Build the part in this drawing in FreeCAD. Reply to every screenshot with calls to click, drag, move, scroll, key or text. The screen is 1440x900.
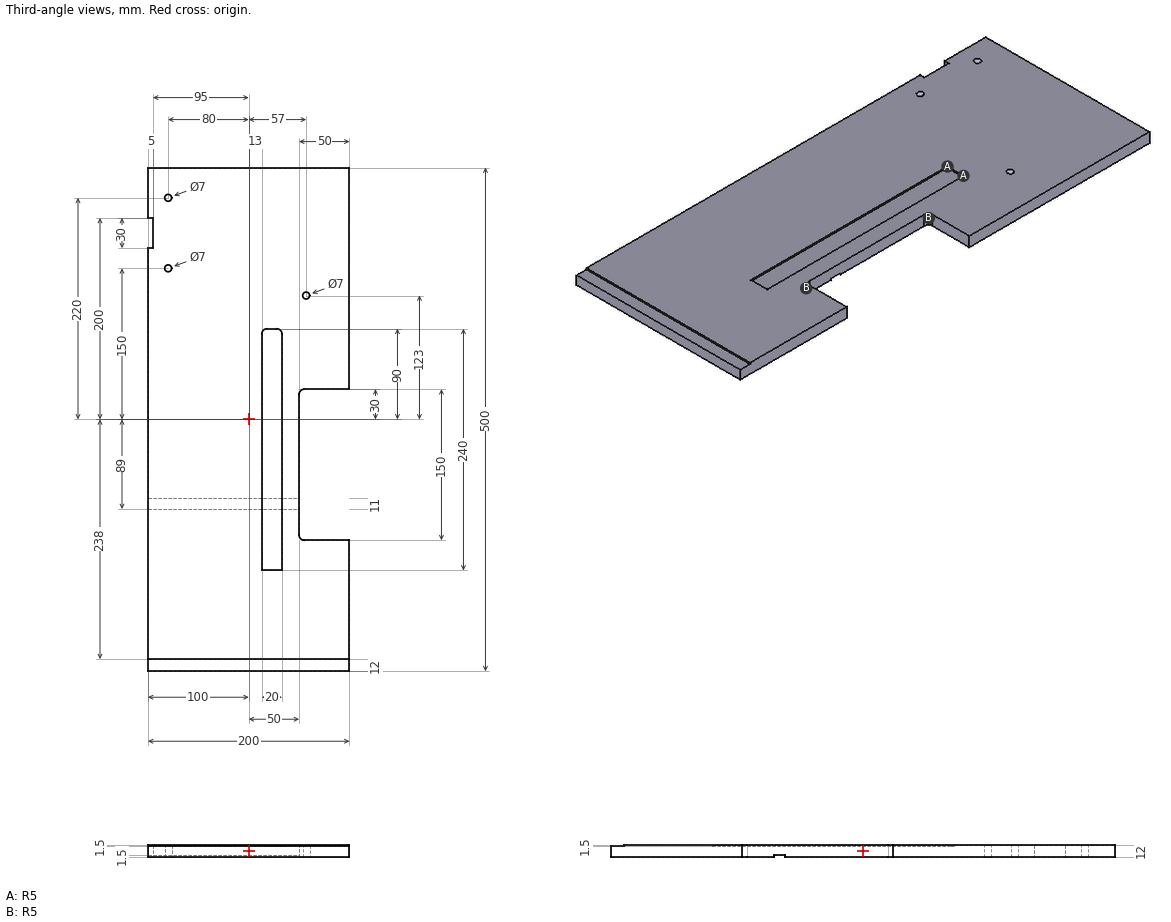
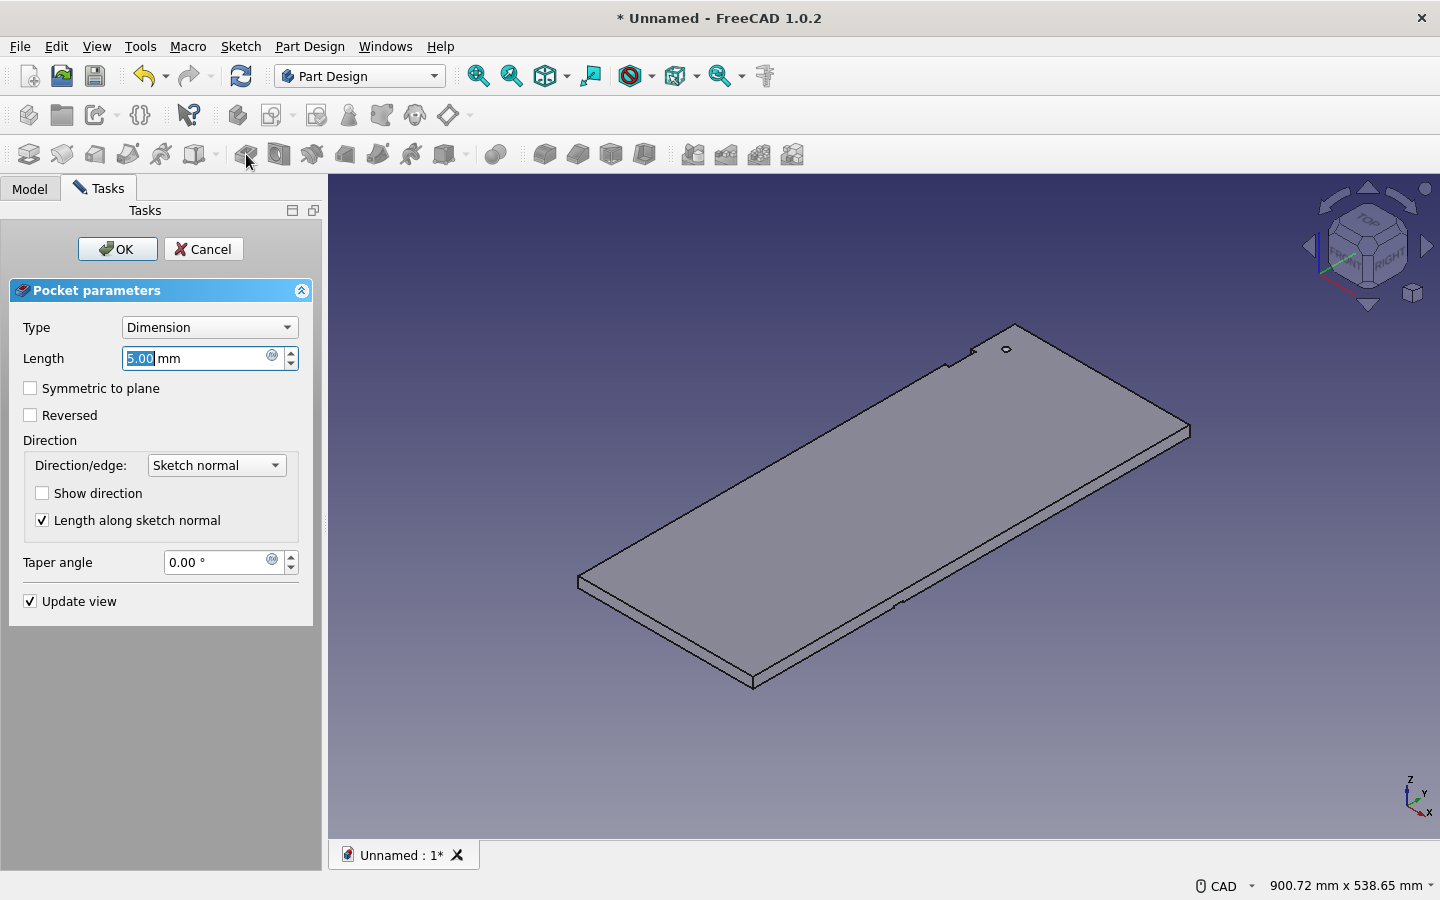
click(210, 328)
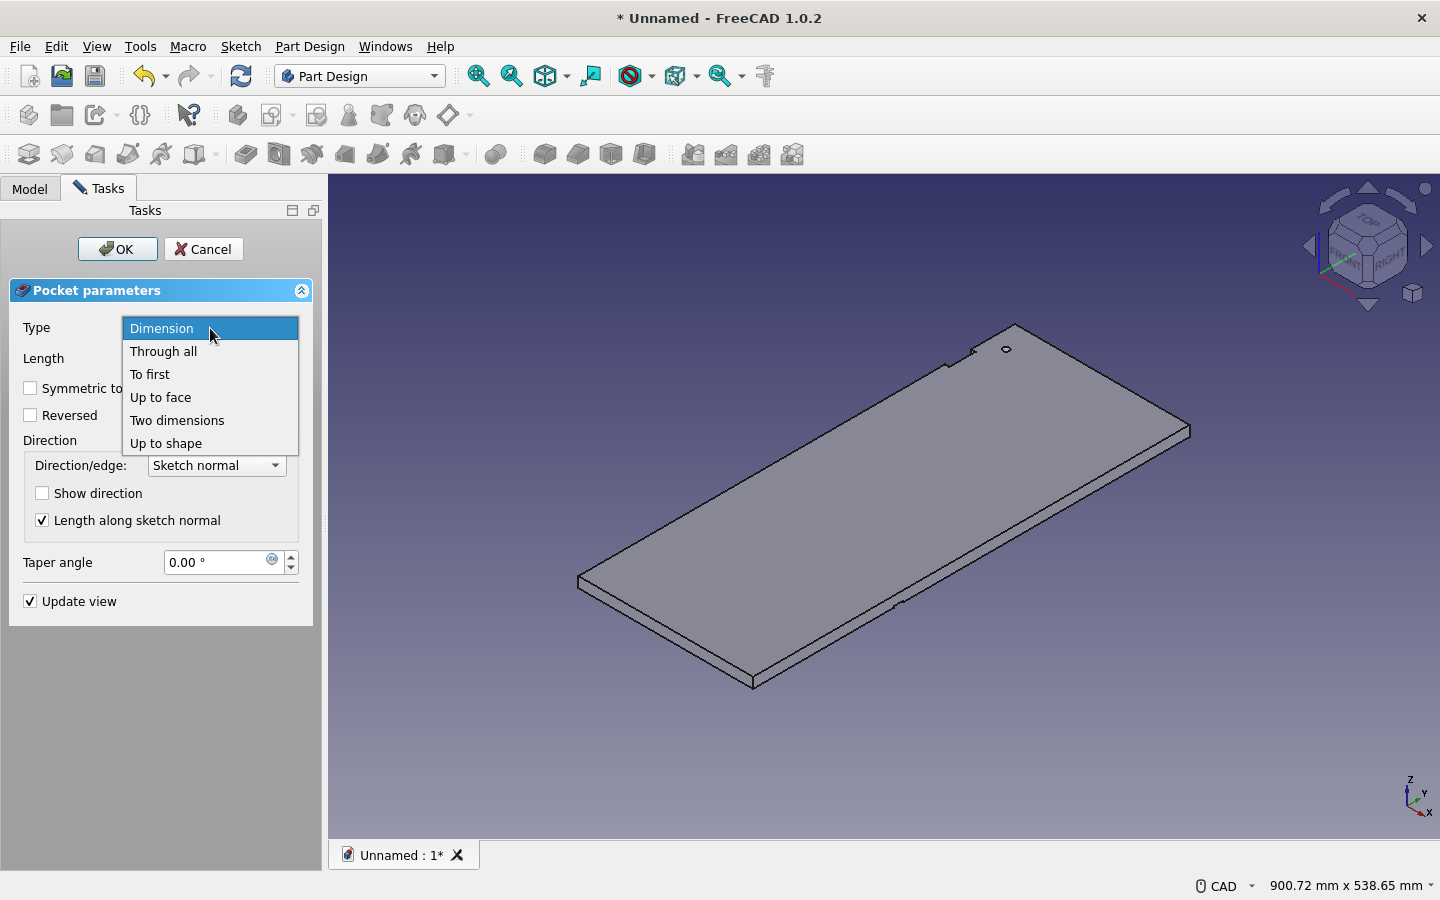
click(208, 374)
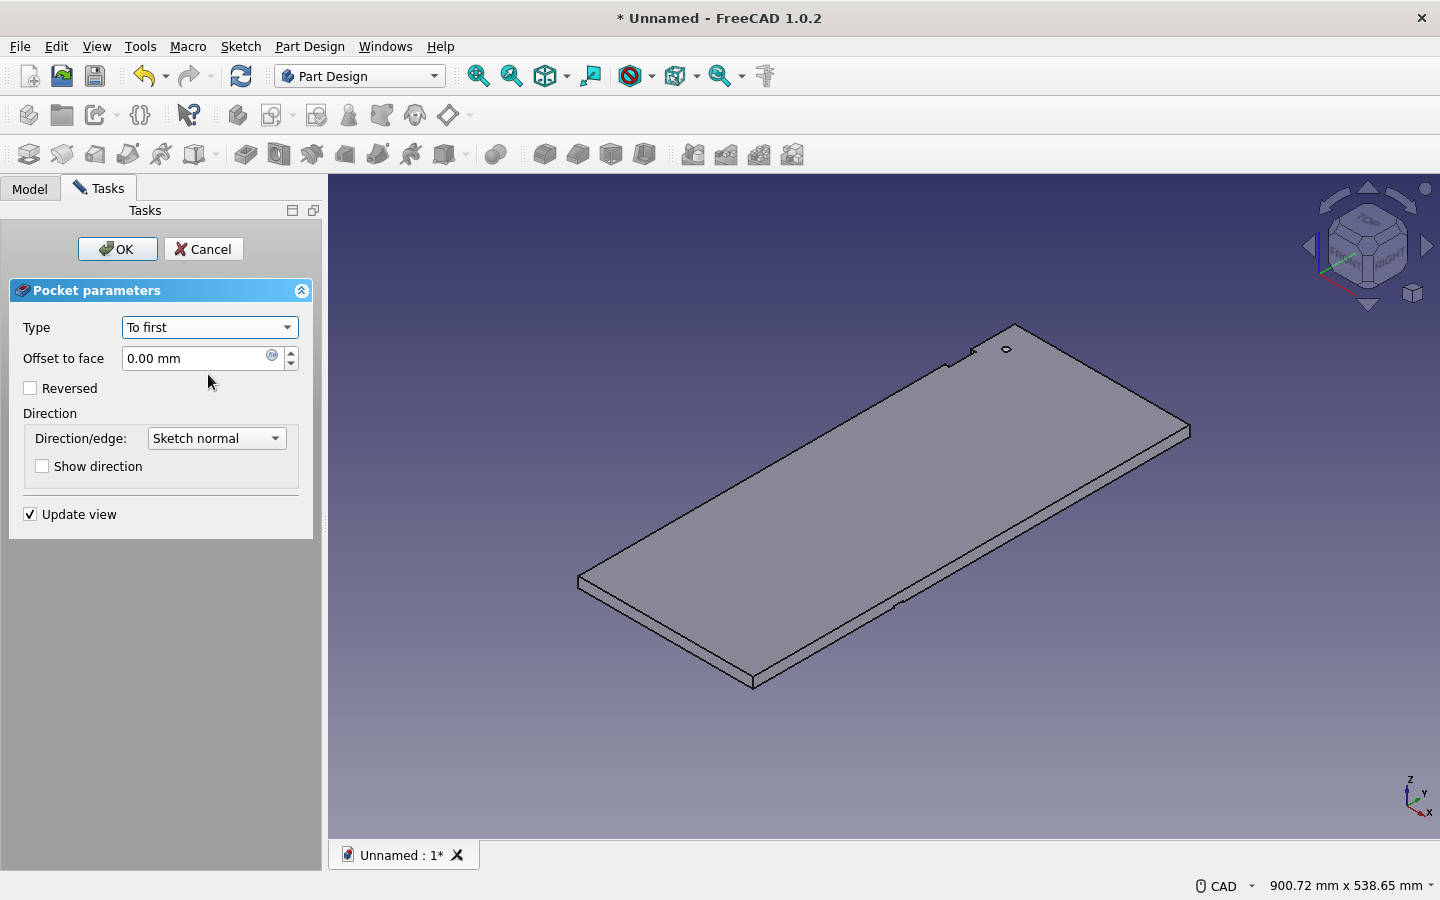
click(118, 249)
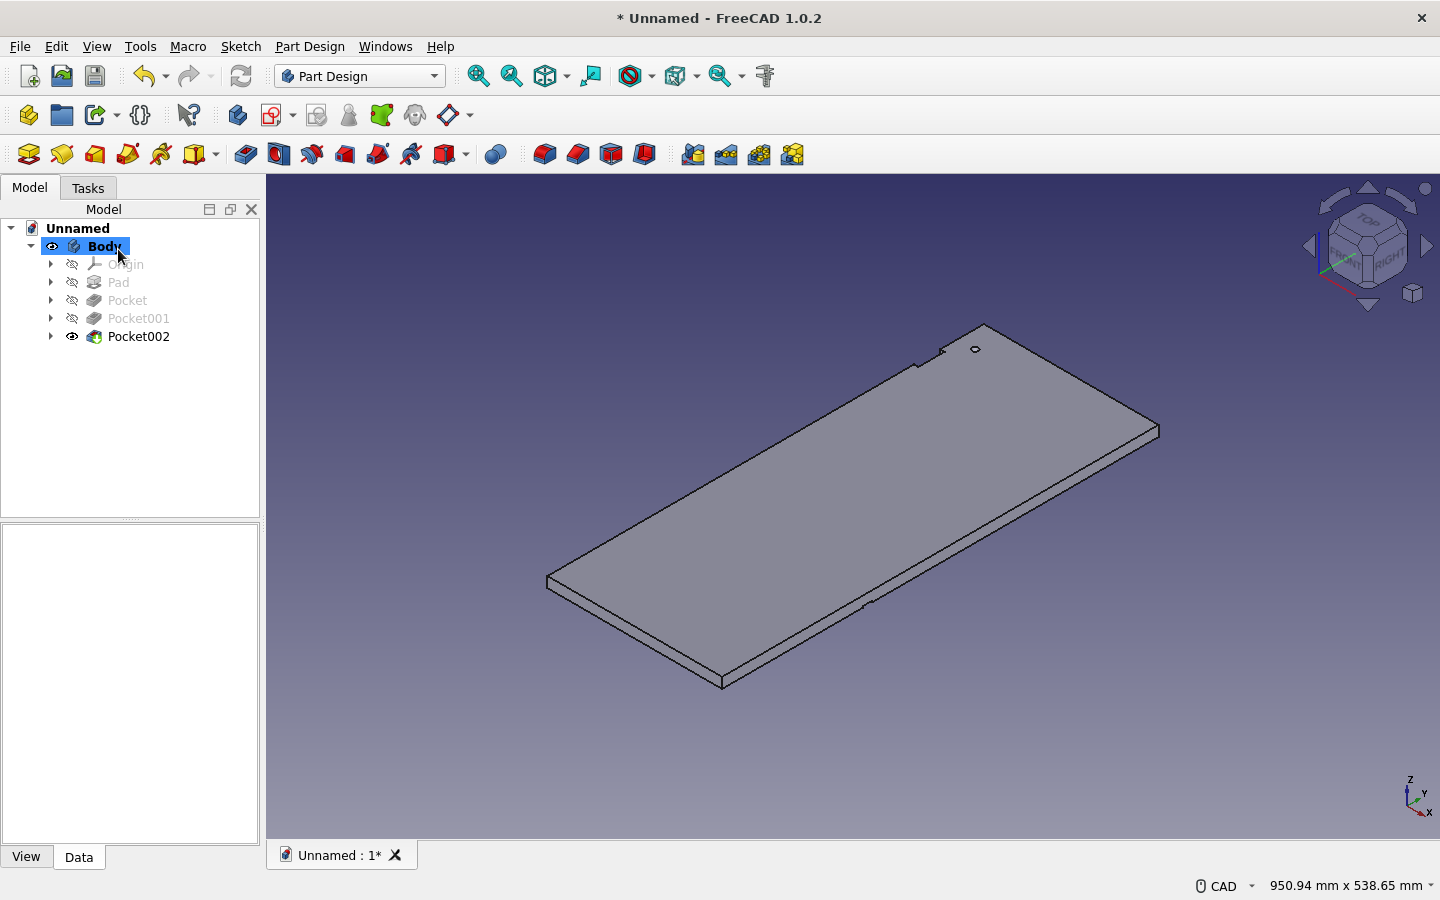
click(915, 463)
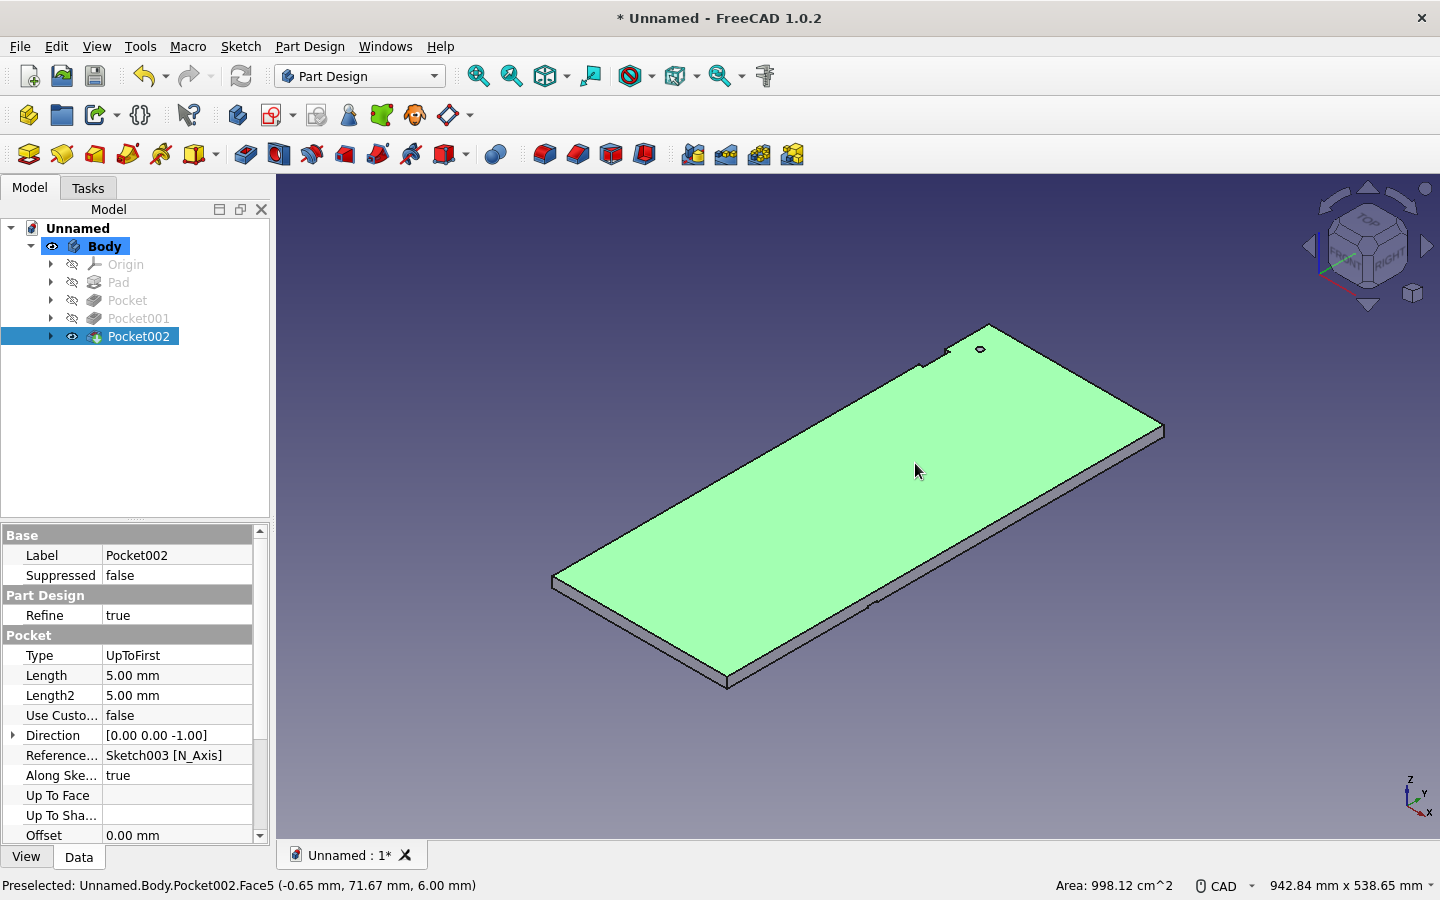
click(270, 116)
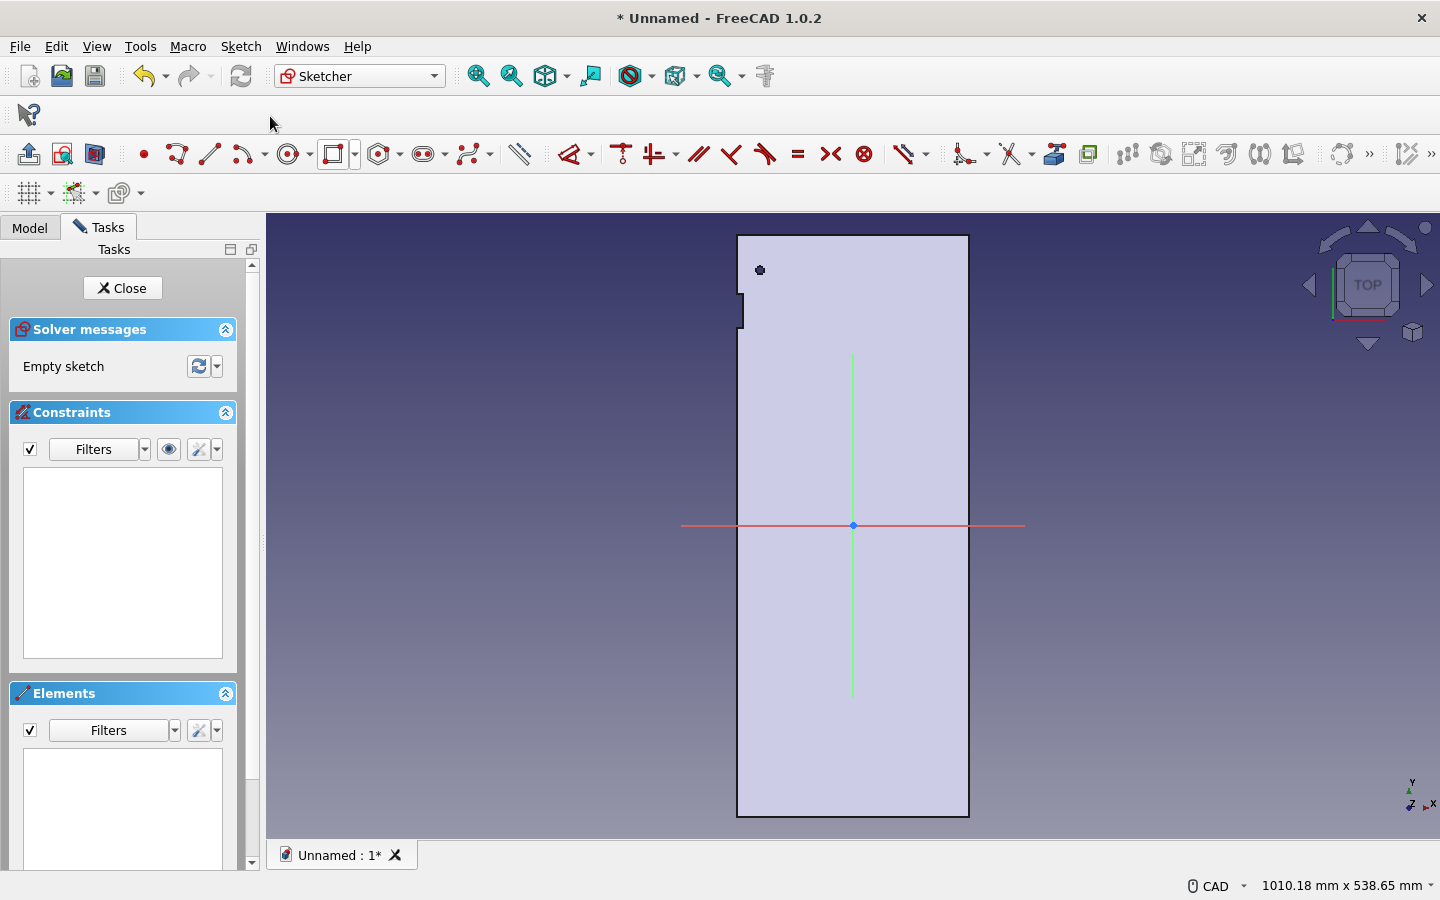
scroll(759, 343, up, 15)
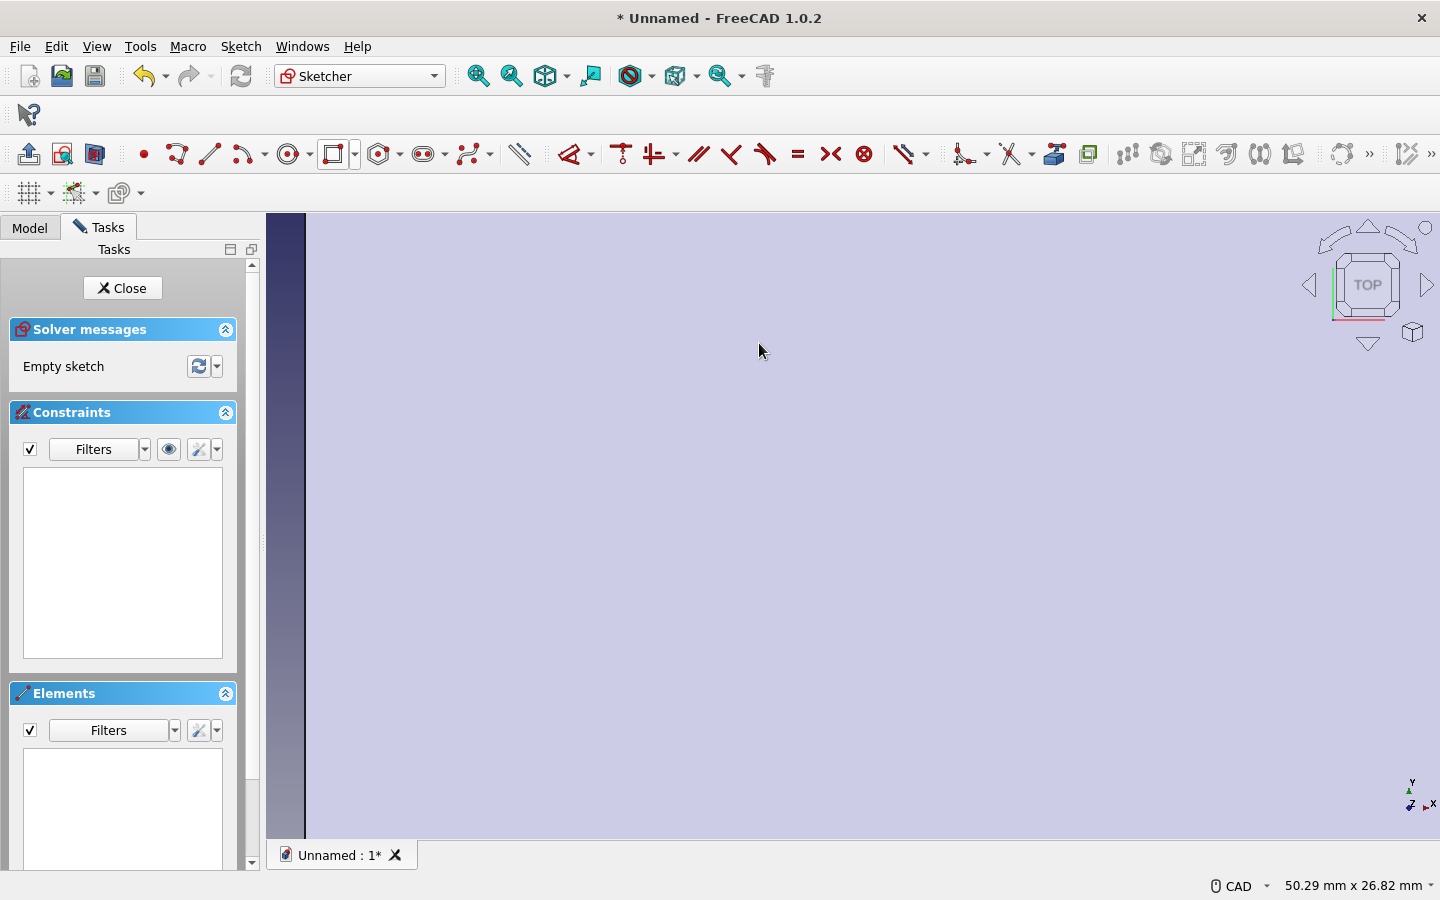
scroll(764, 506, up, 5)